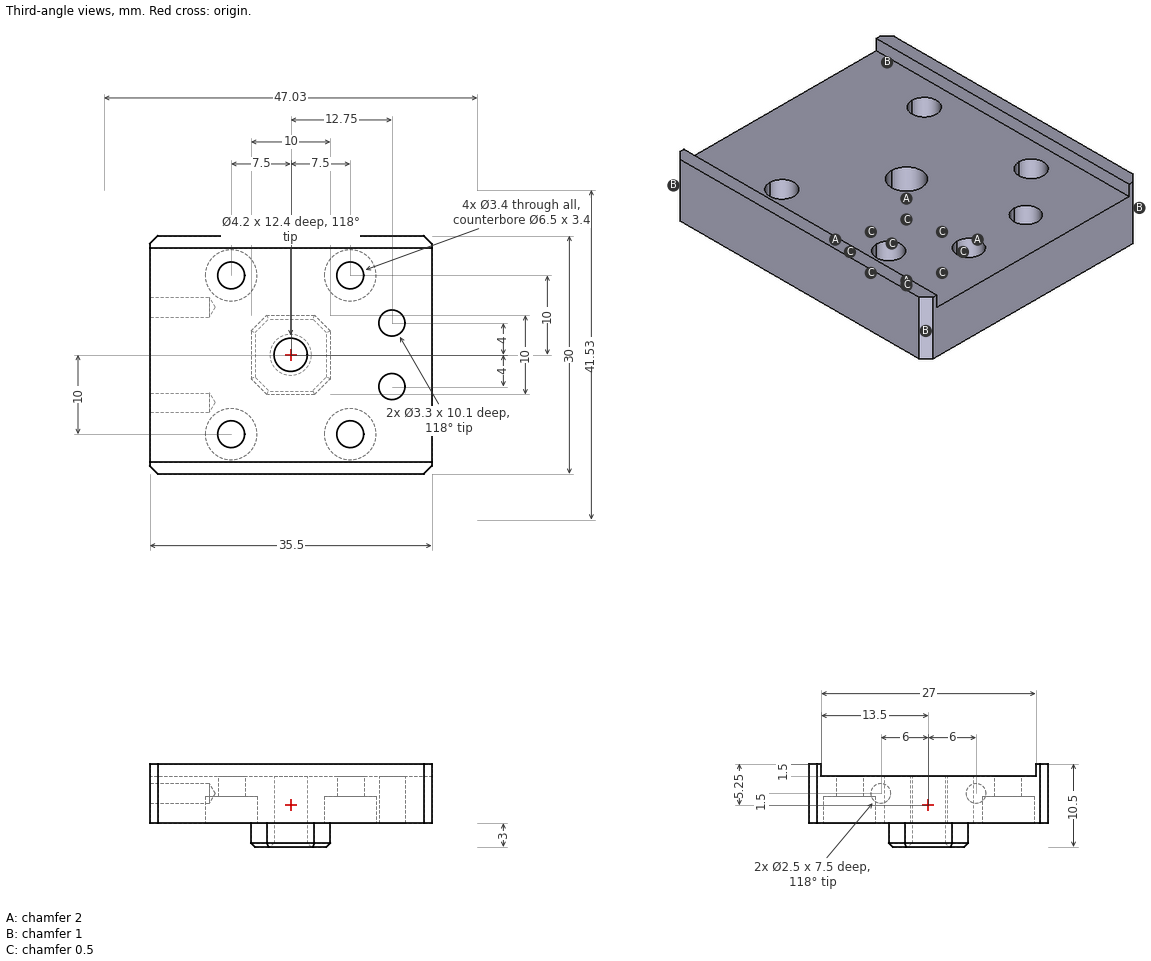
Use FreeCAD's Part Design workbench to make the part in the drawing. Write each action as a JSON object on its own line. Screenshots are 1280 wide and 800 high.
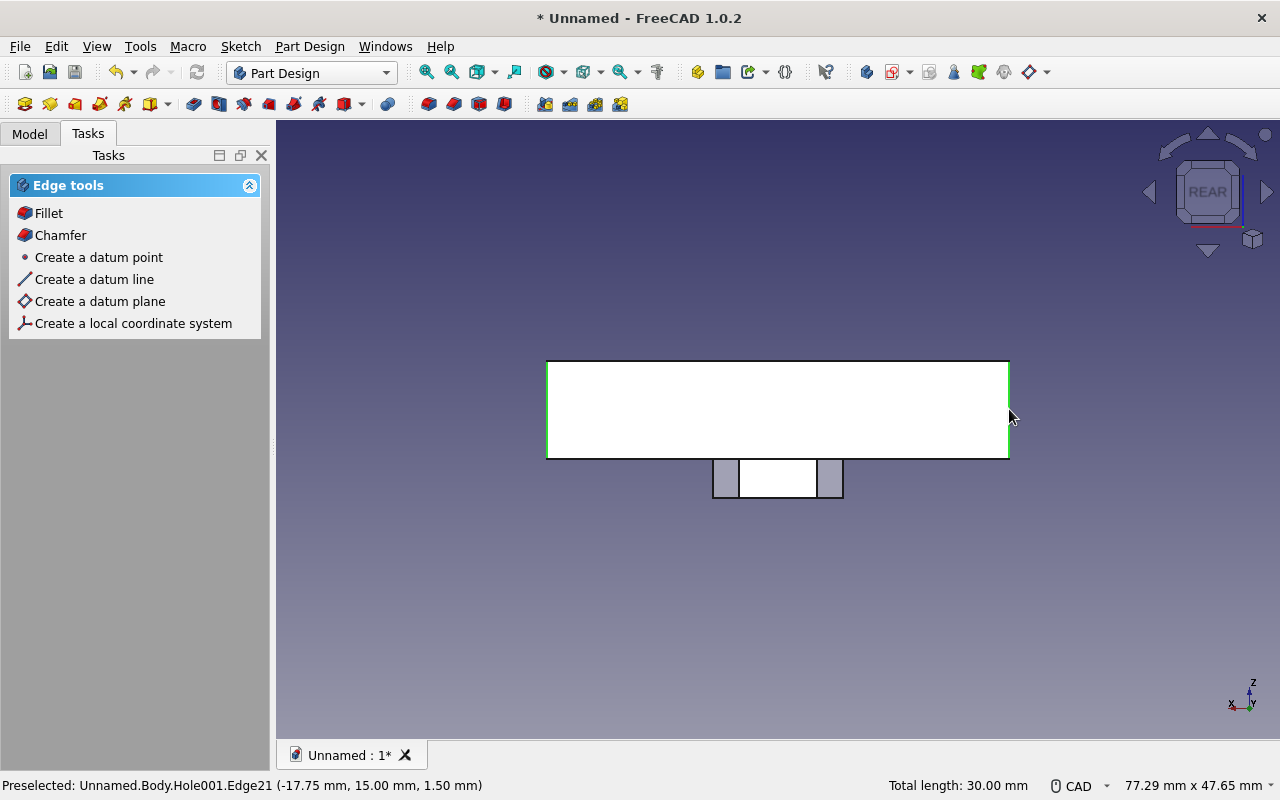
{"action": "left_click", "coordinate": [454, 104]}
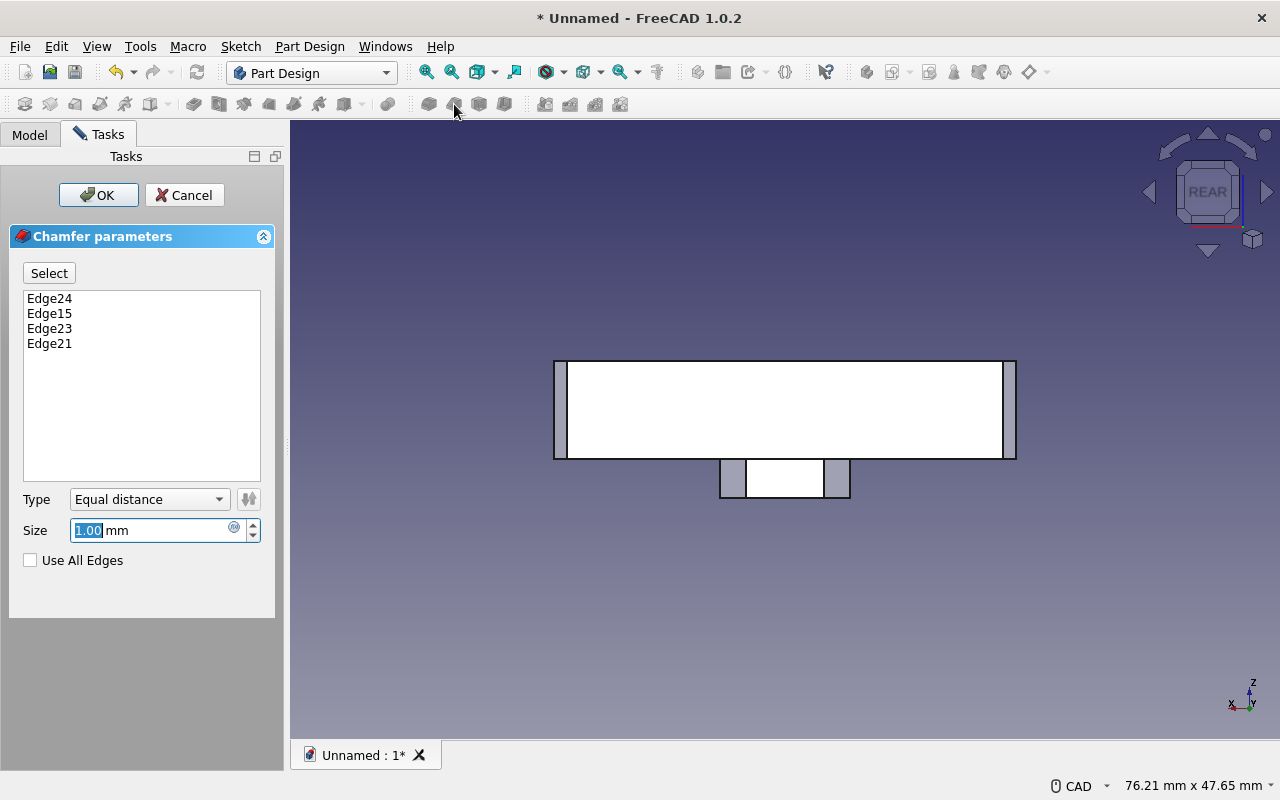
{"action": "type", "text": "1"}
{"action": "key", "text": "Tab"}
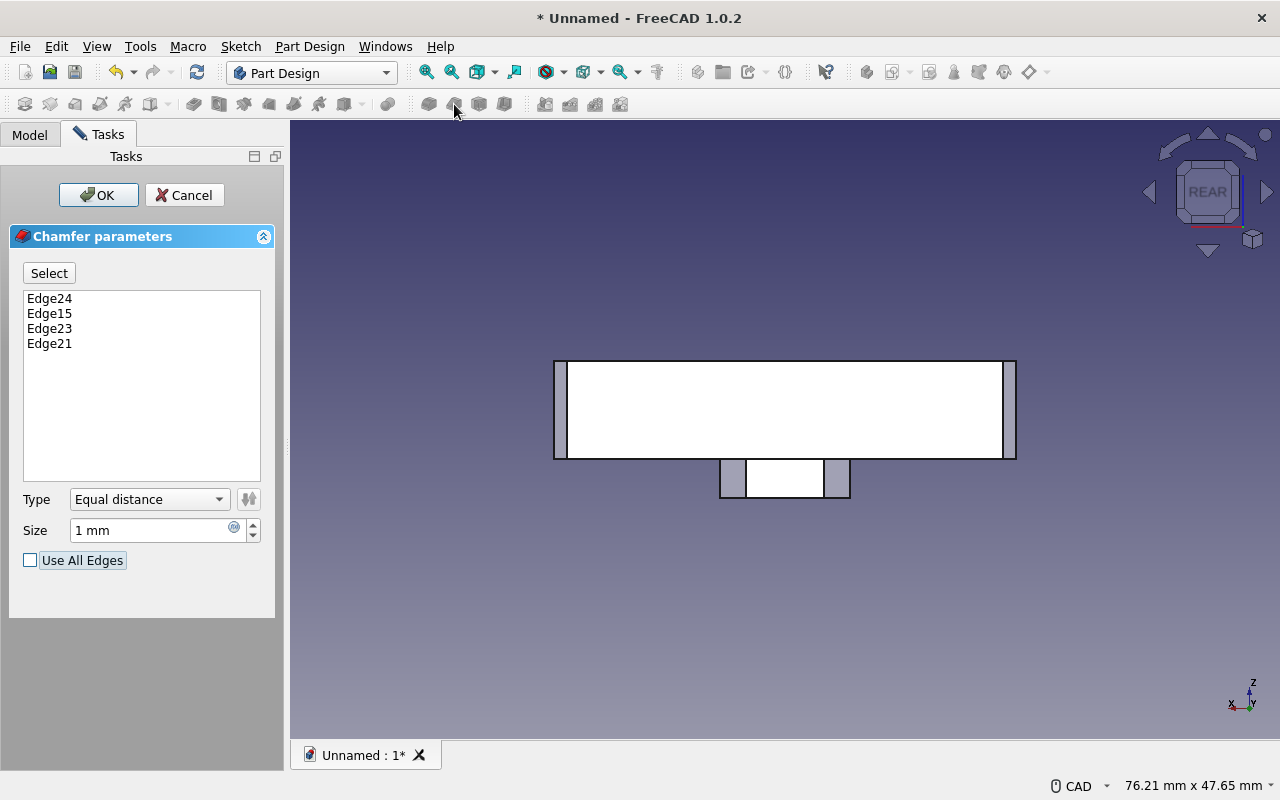
{"action": "left_click", "coordinate": [99, 195]}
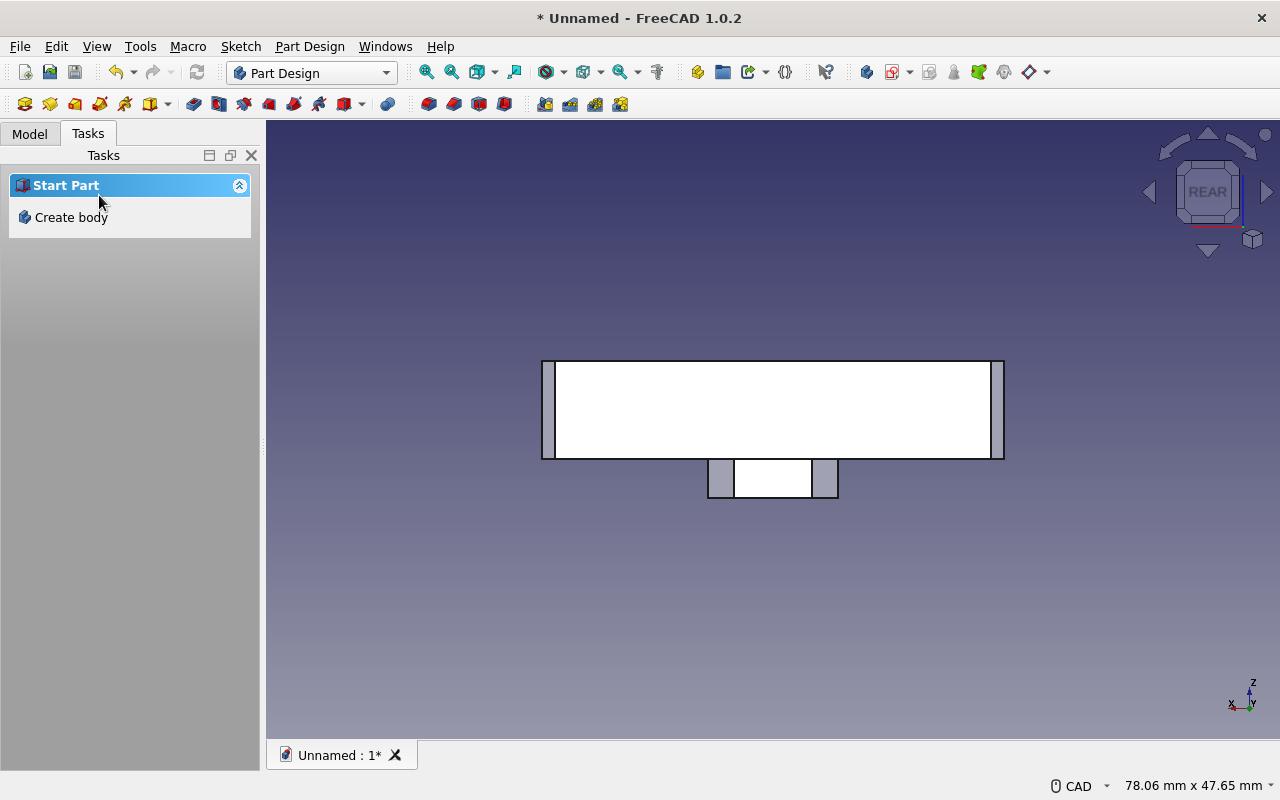
{"action": "key", "text": "0"}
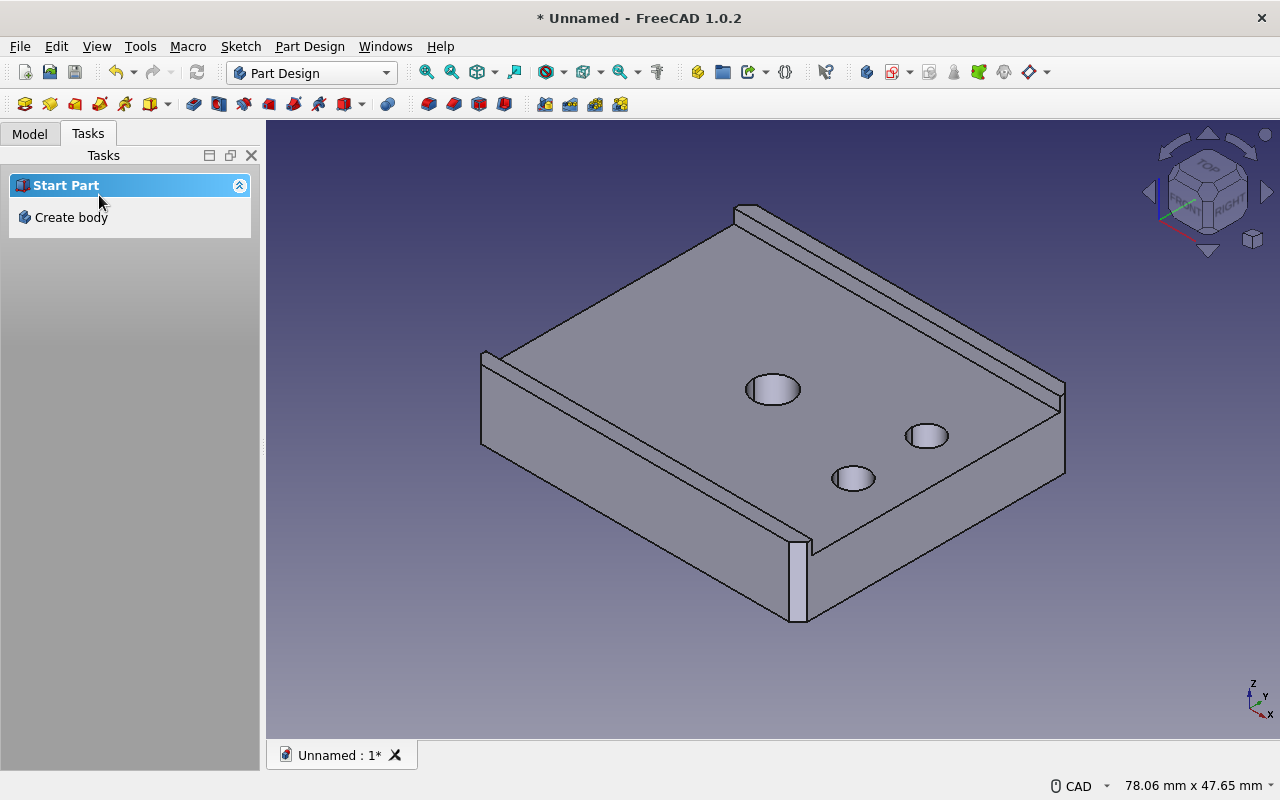
{"action": "key", "text": "2"}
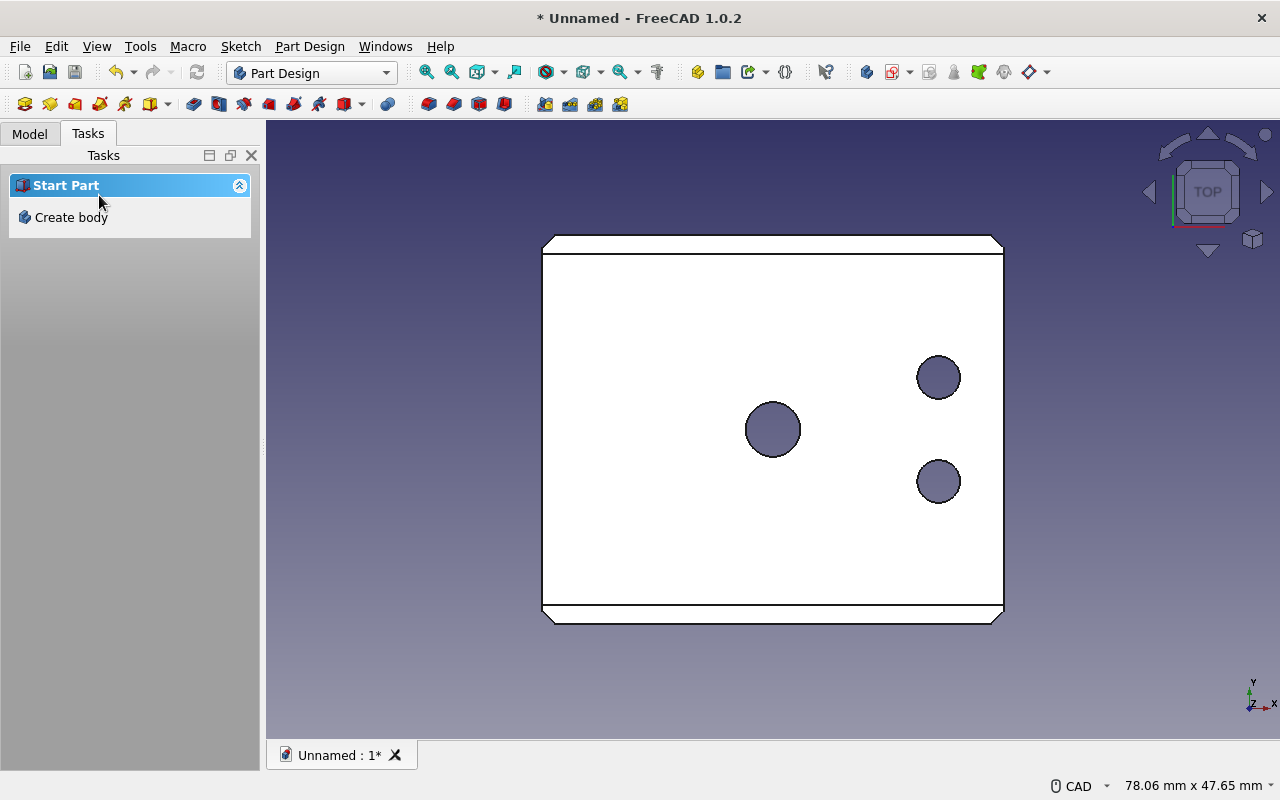
{"action": "key", "text": "1"}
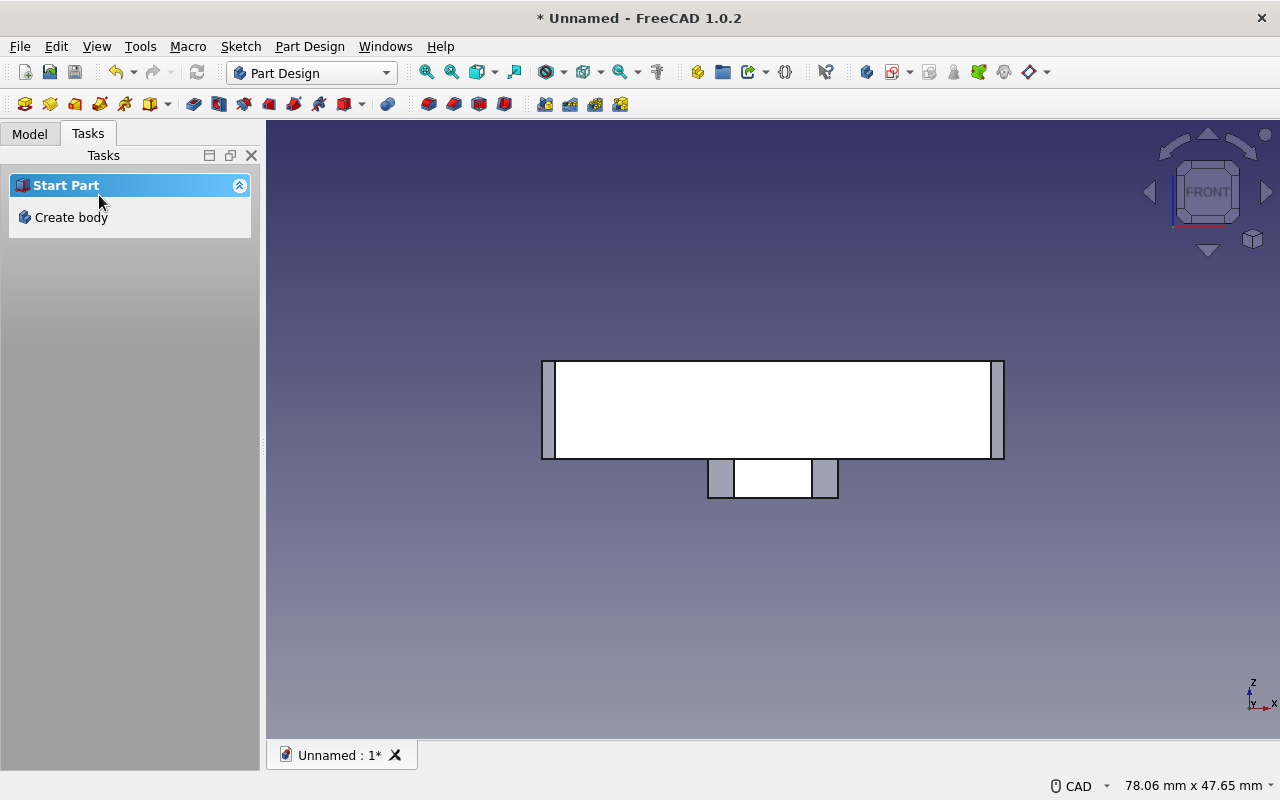
{"action": "key", "text": "3"}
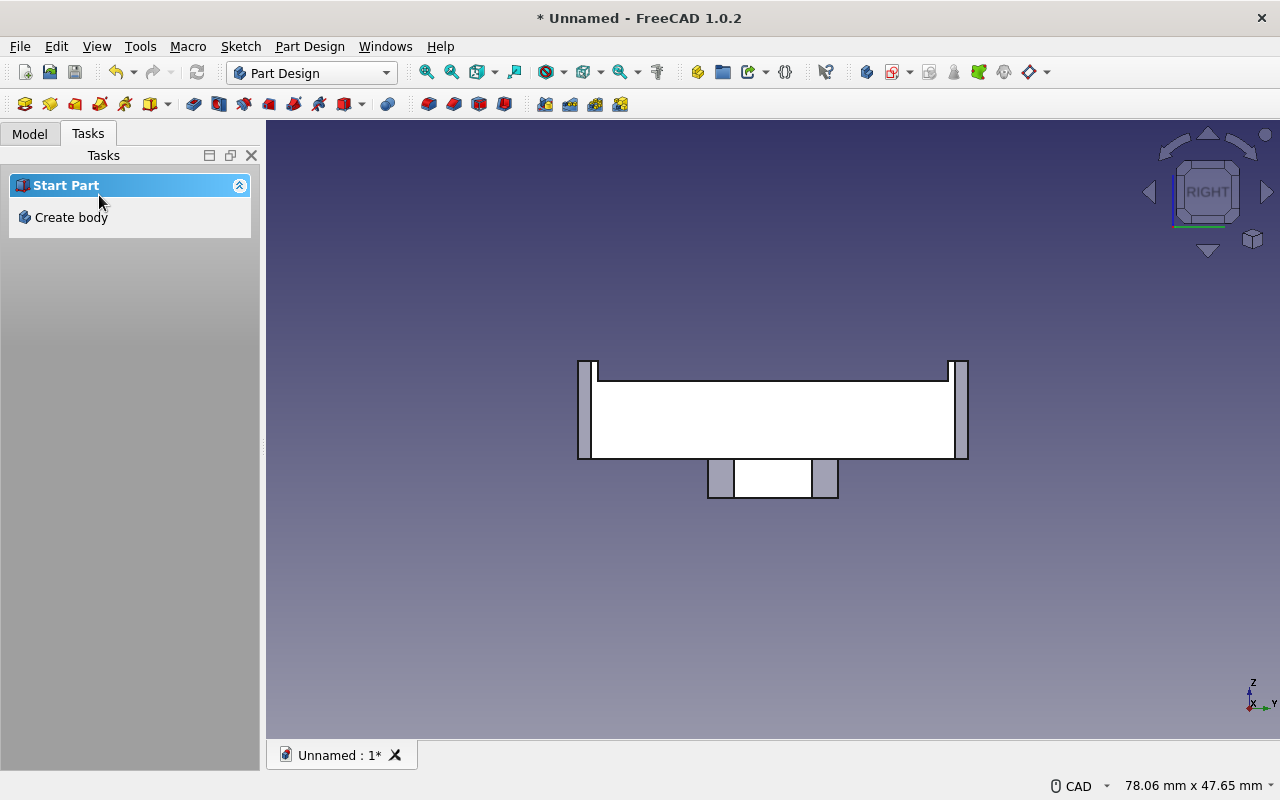
{"action": "key", "text": "v f"}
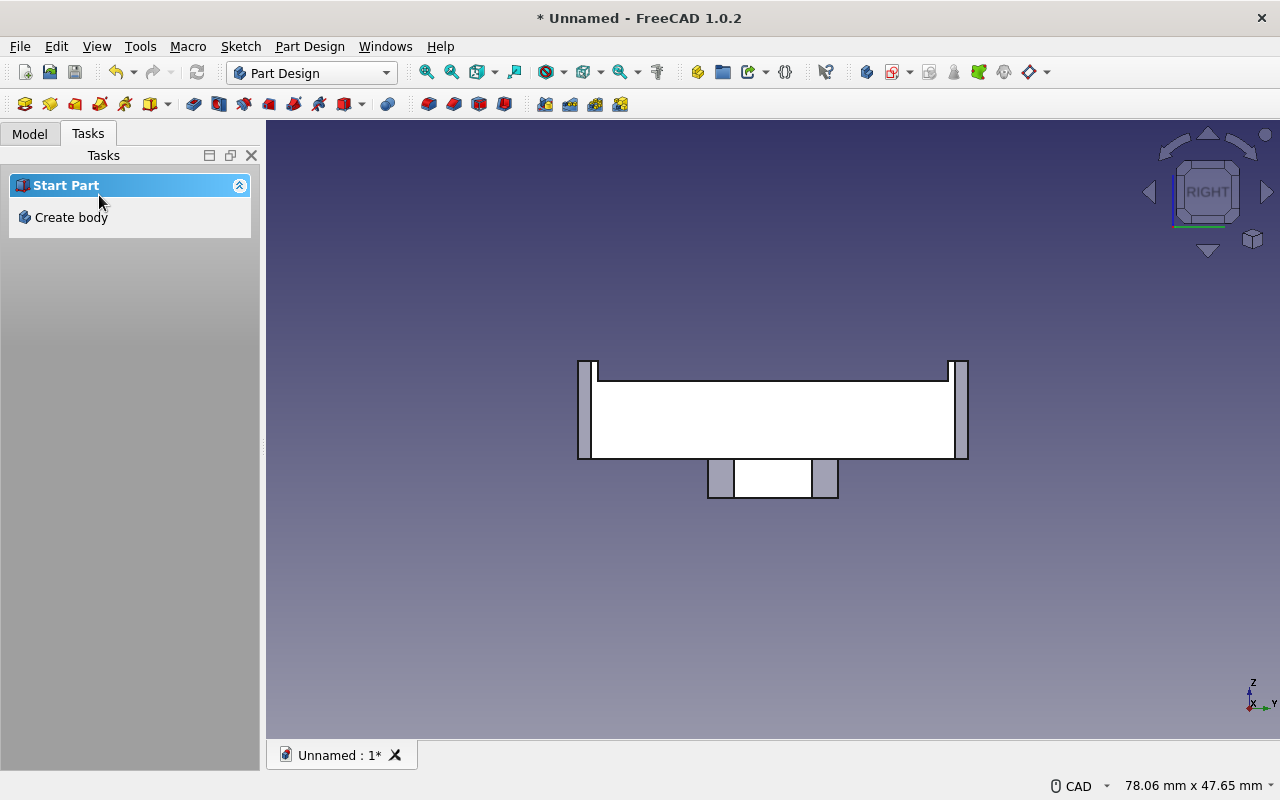
{"action": "key", "text": "5"}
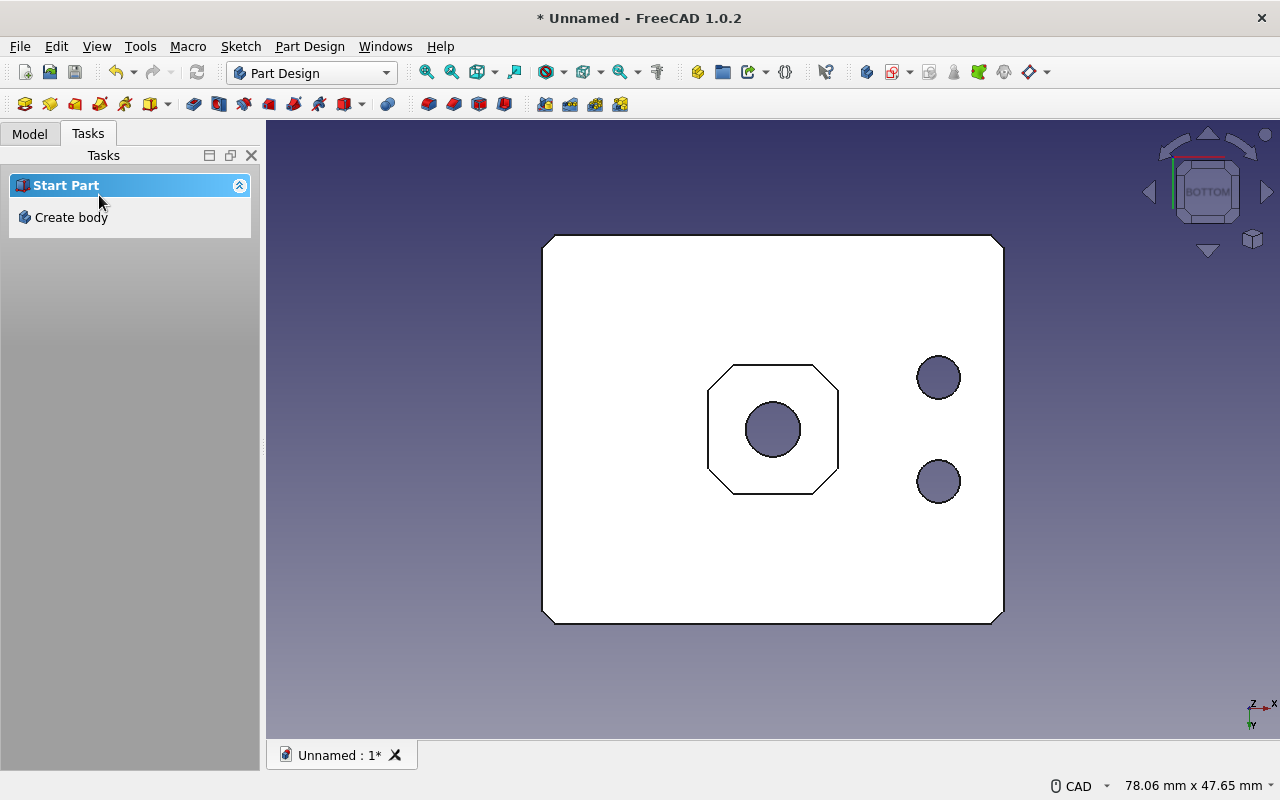
{"action": "left_click", "coordinate": [810, 466]}